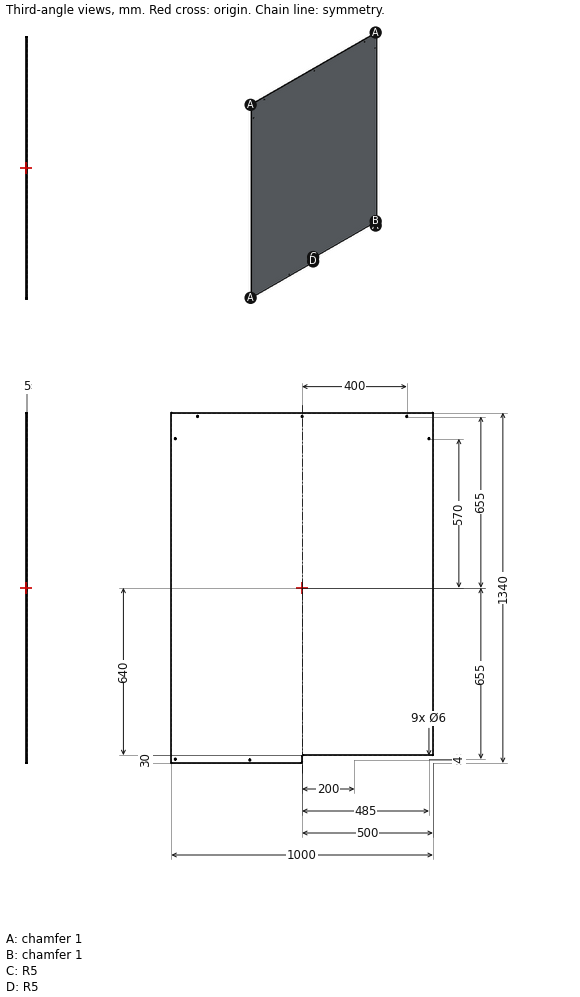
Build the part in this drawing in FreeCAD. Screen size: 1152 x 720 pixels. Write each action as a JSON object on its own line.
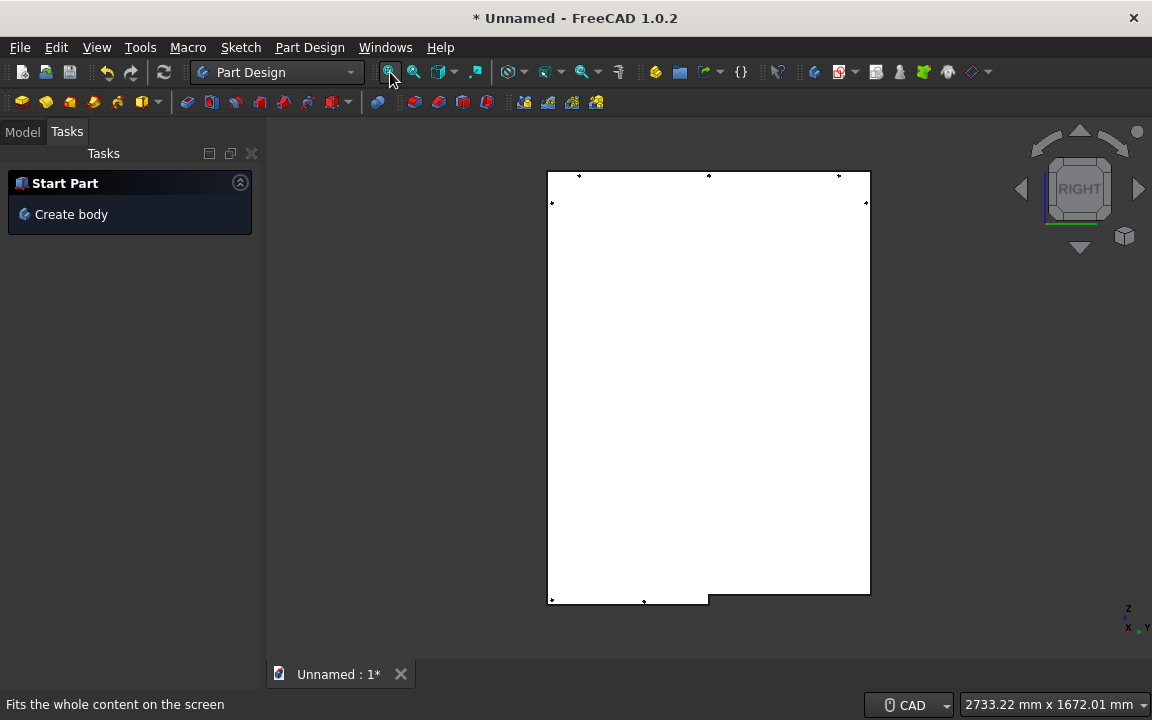
{"action": "scroll", "coordinate": [871, 594], "scroll_direction": "up", "scroll_amount": 15}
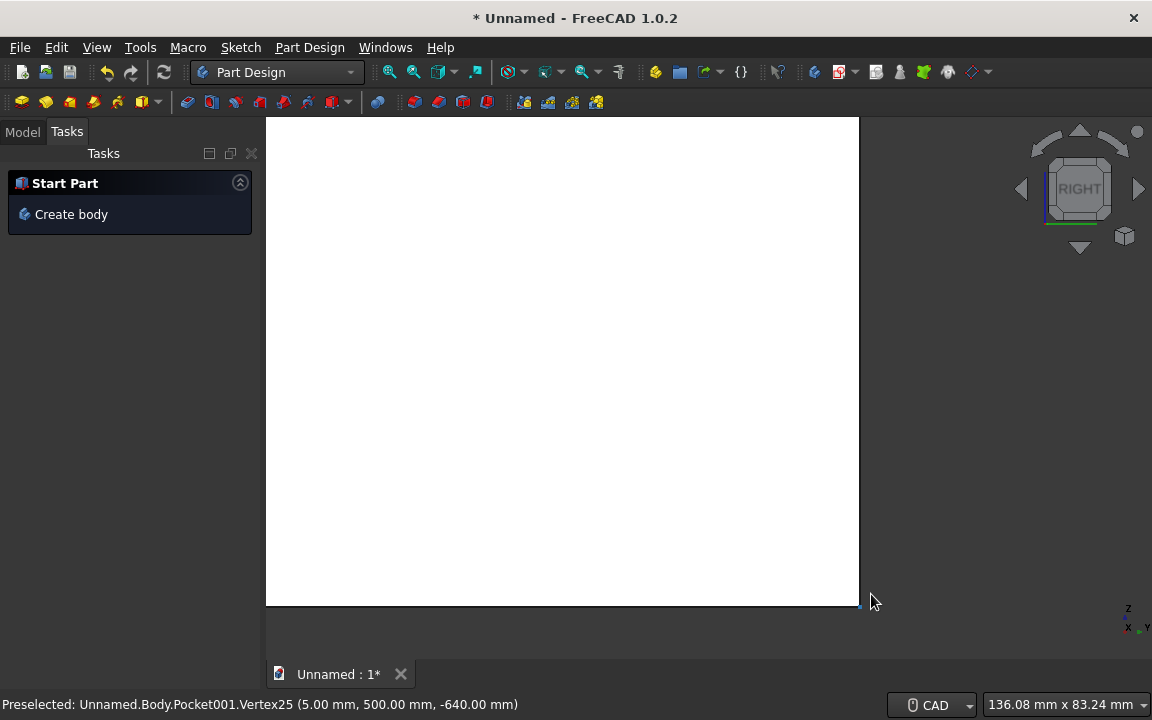
{"action": "left_click", "coordinate": [390, 72]}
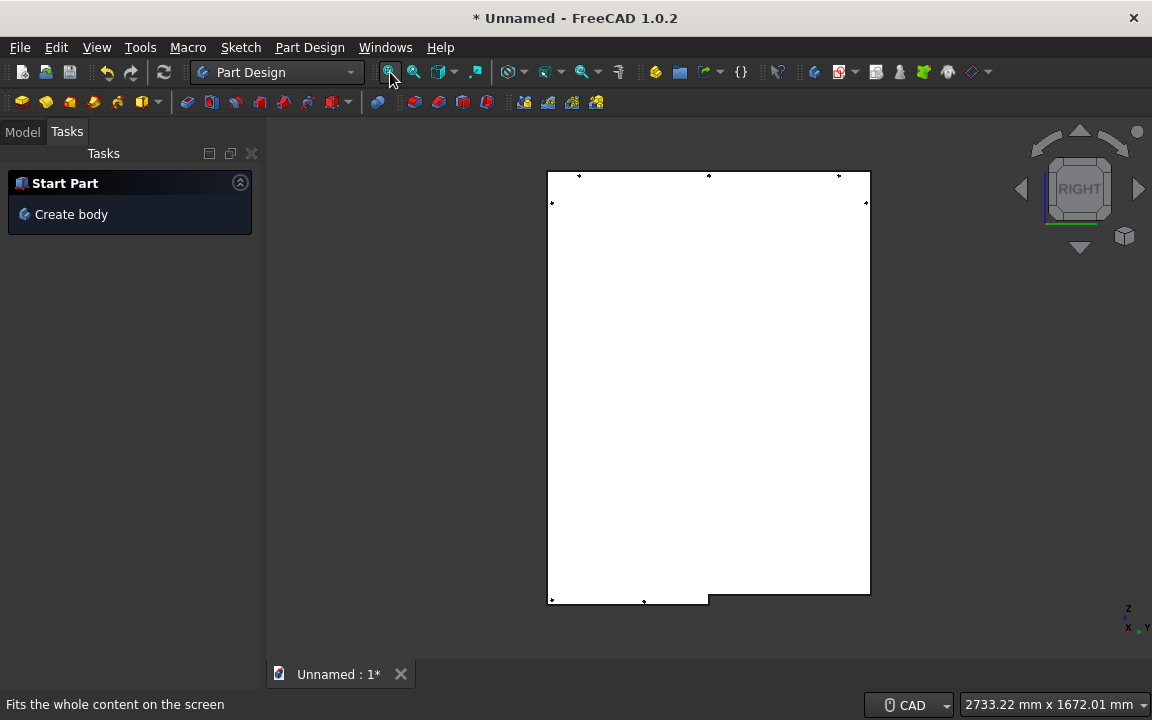
{"action": "key", "text": "5"}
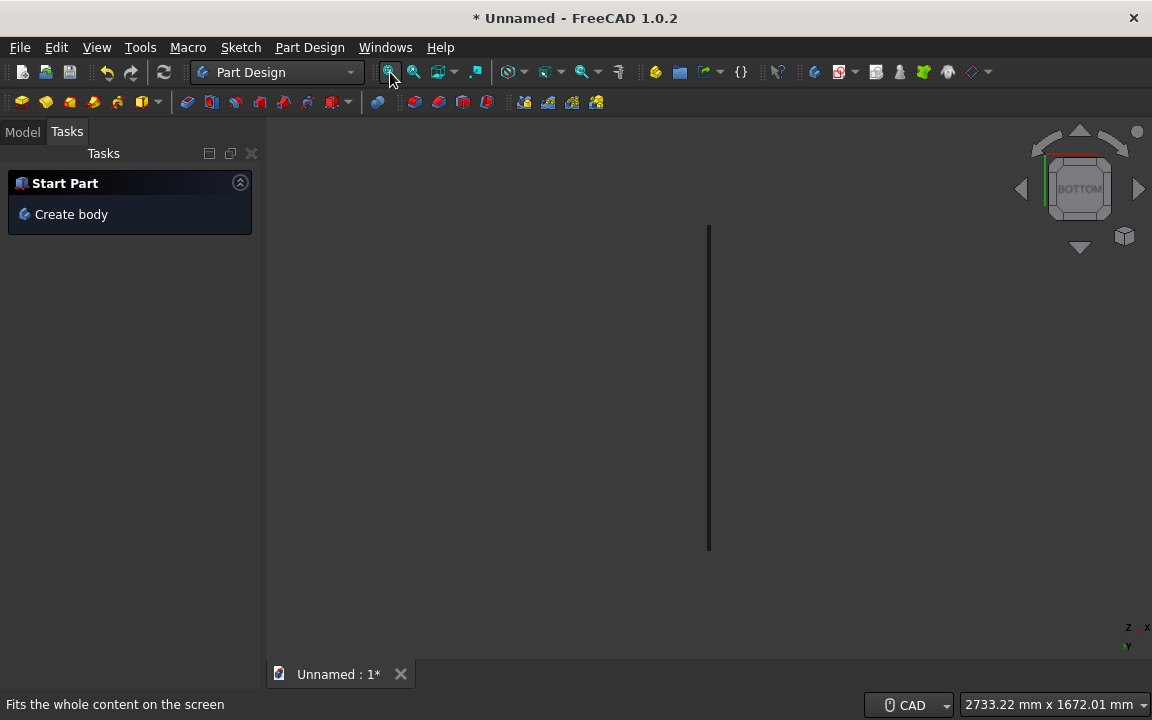
{"action": "scroll", "coordinate": [709, 549], "scroll_direction": "up", "scroll_amount": 15}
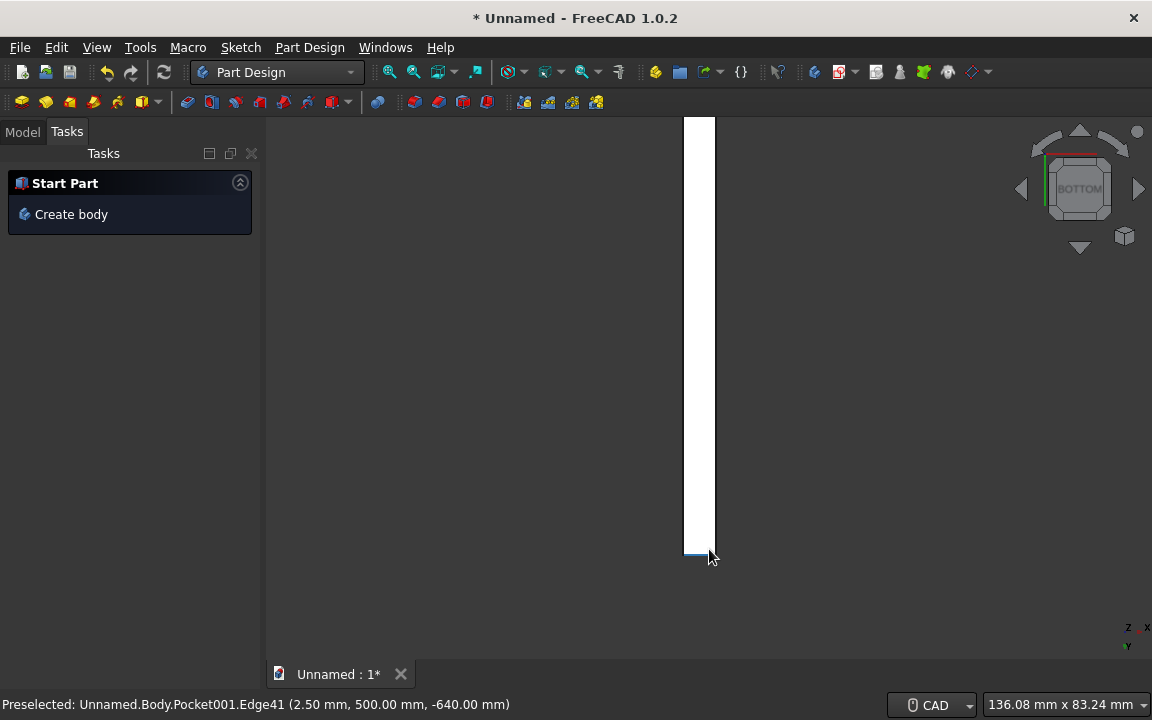
{"action": "left_click", "coordinate": [699, 554]}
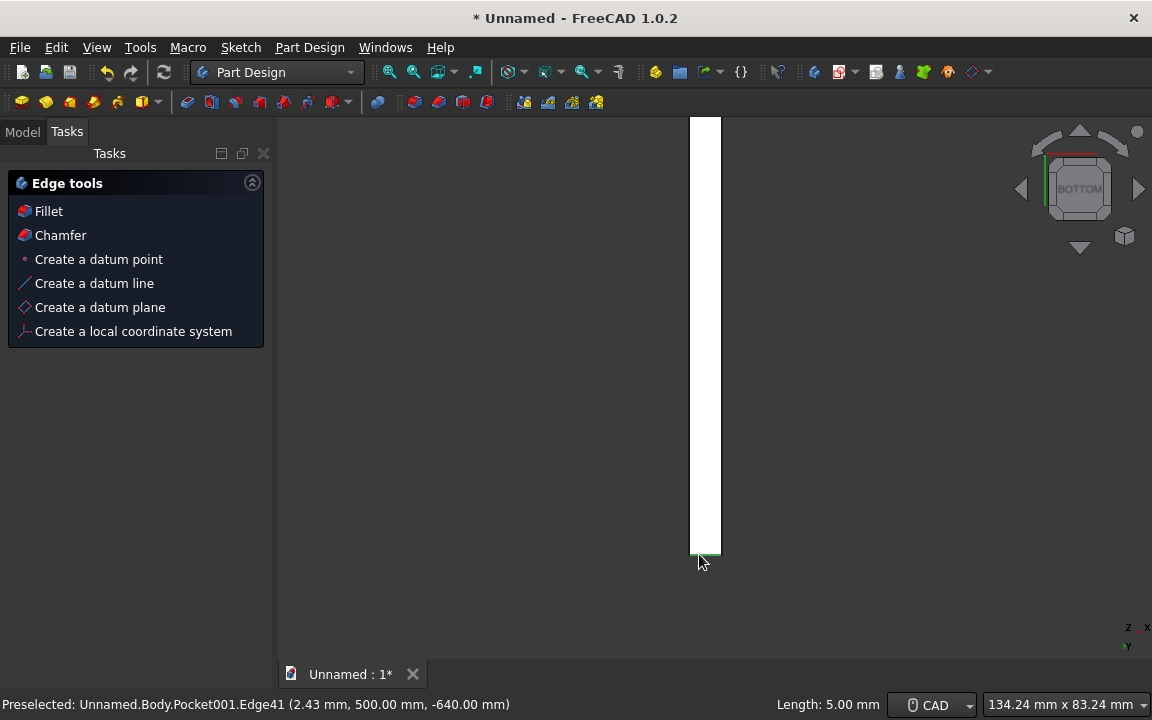
{"action": "left_click", "coordinate": [440, 102]}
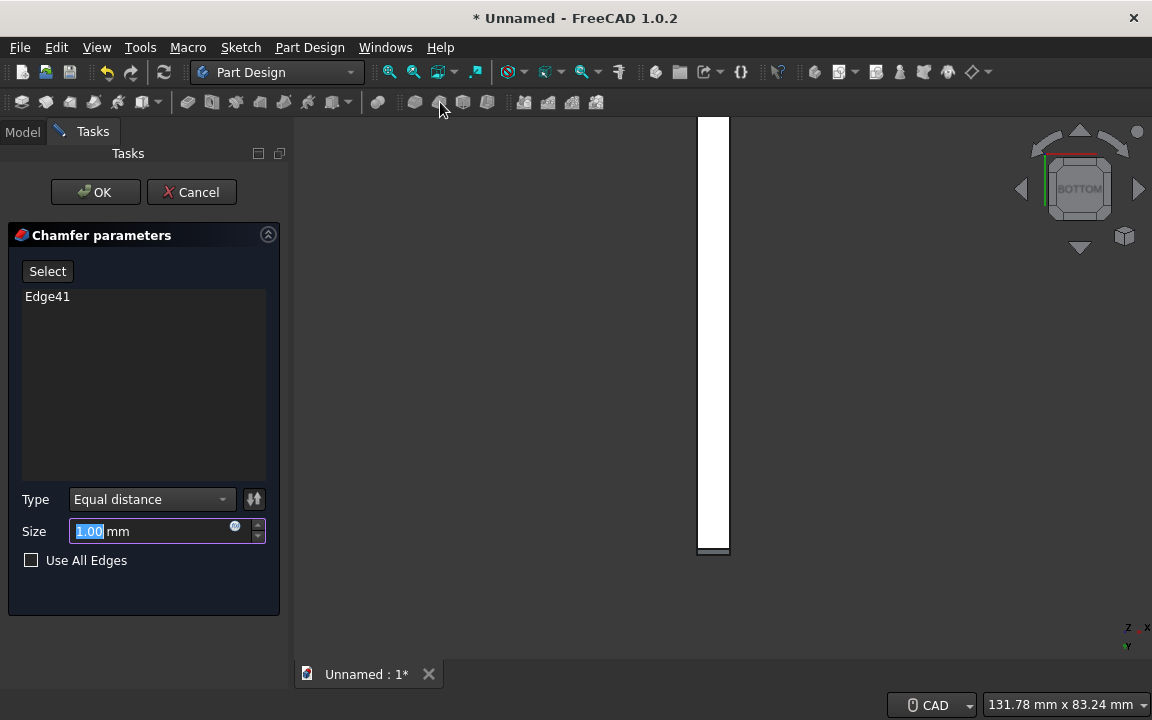
{"action": "type", "text": "1"}
{"action": "key", "text": "Tab"}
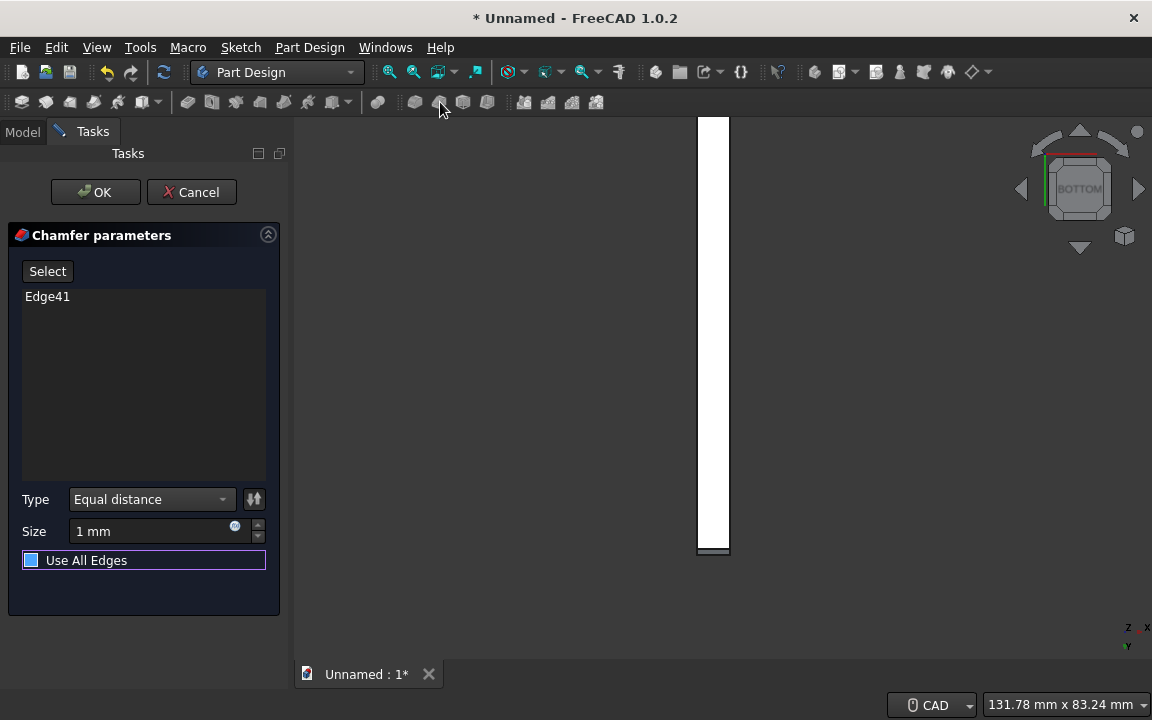
{"action": "left_click", "coordinate": [96, 192]}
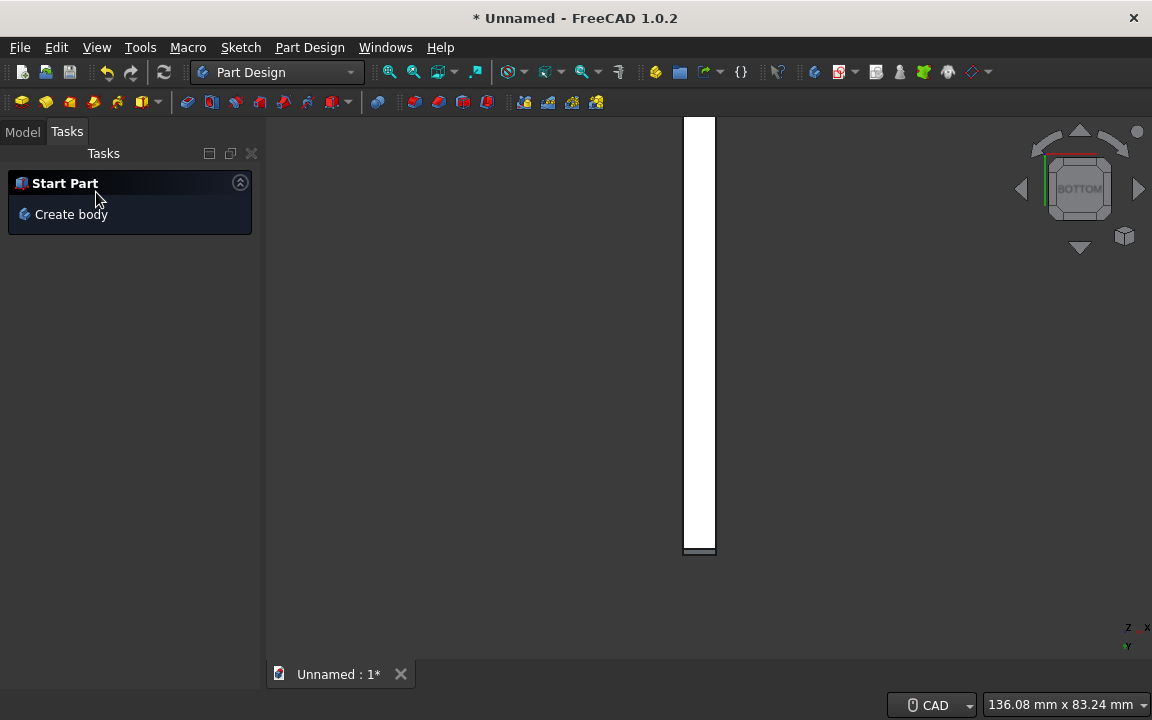
{"action": "left_click", "coordinate": [390, 72]}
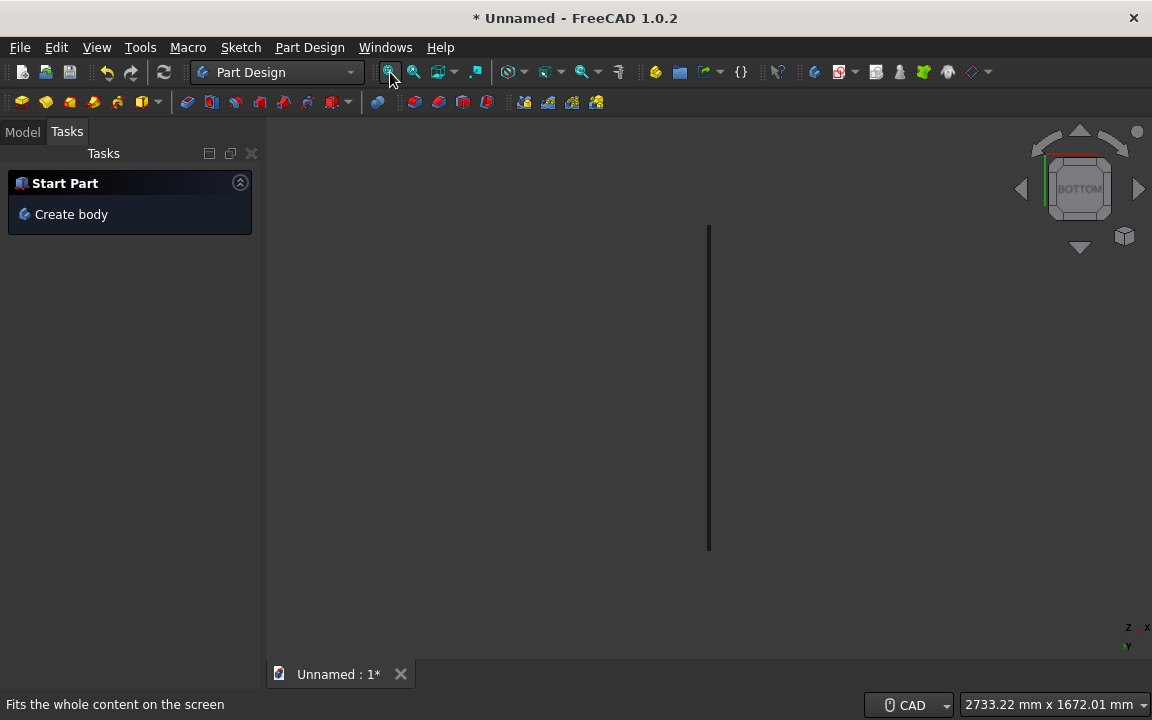
{"action": "scroll", "coordinate": [709, 387], "scroll_direction": "up", "scroll_amount": 15}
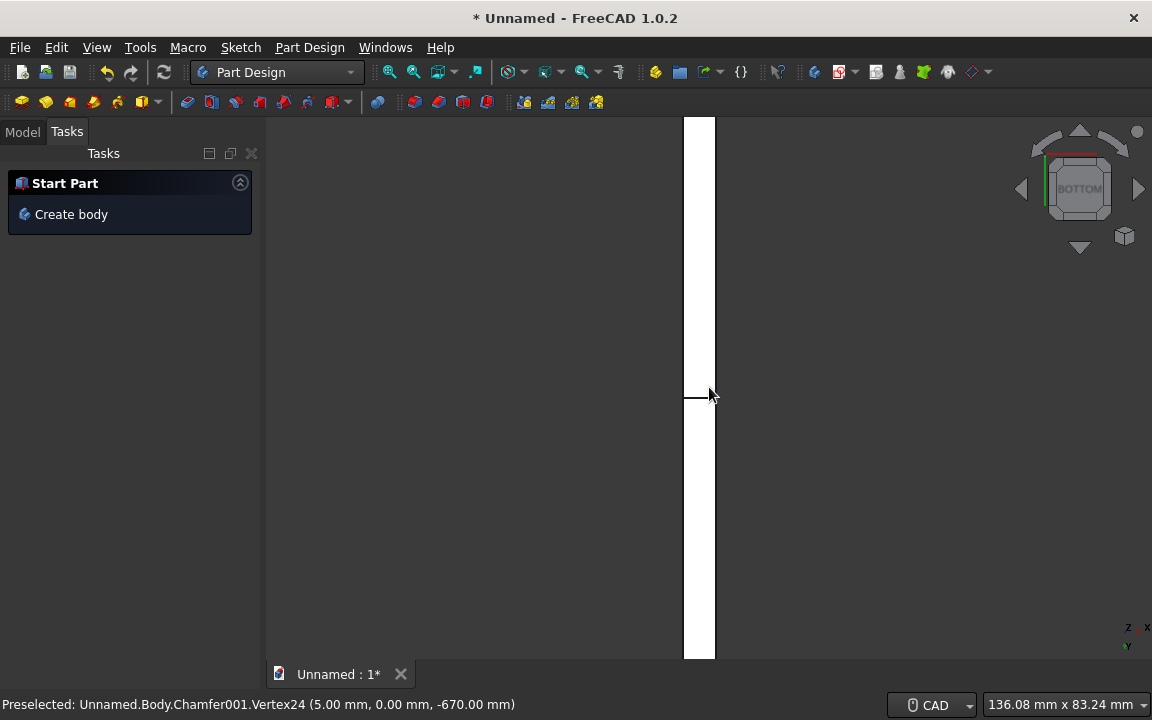
{"action": "left_click", "coordinate": [390, 72]}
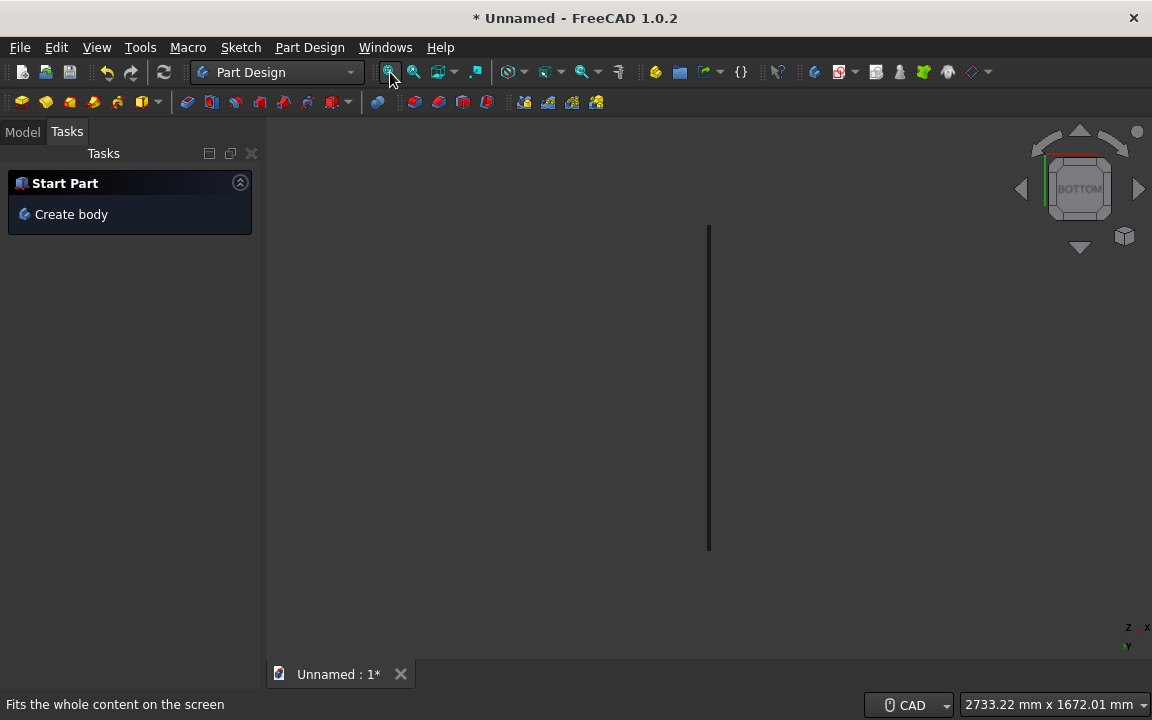
{"action": "key", "text": "0"}